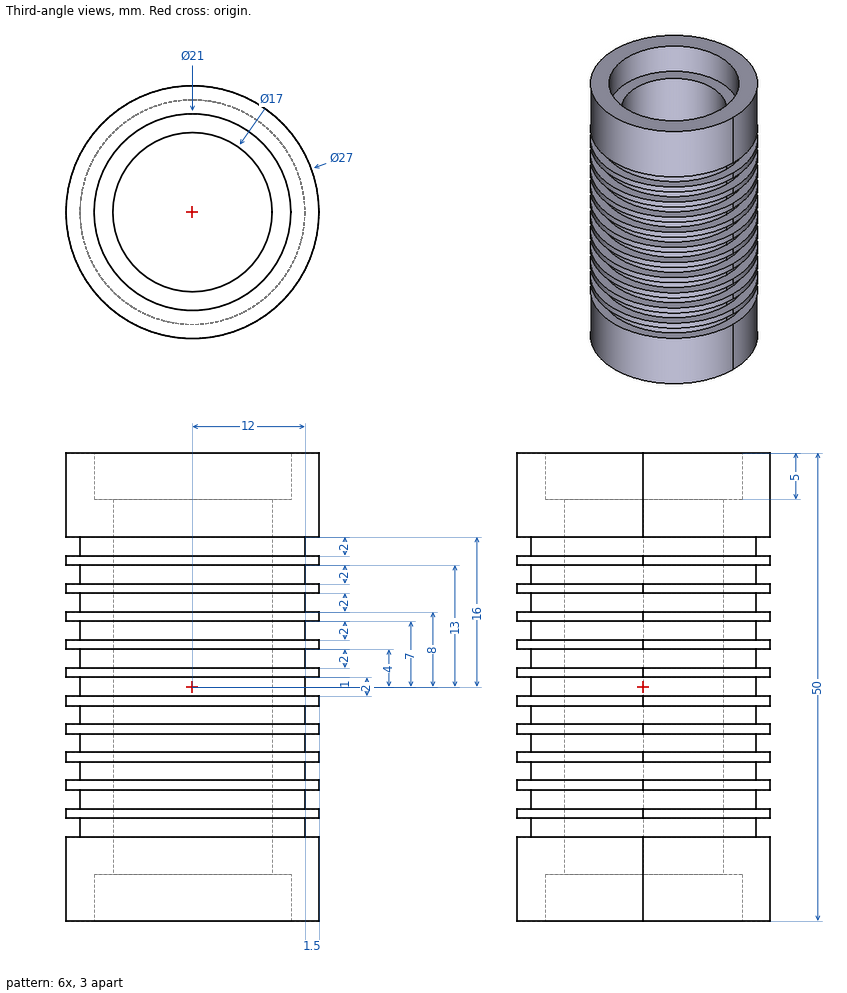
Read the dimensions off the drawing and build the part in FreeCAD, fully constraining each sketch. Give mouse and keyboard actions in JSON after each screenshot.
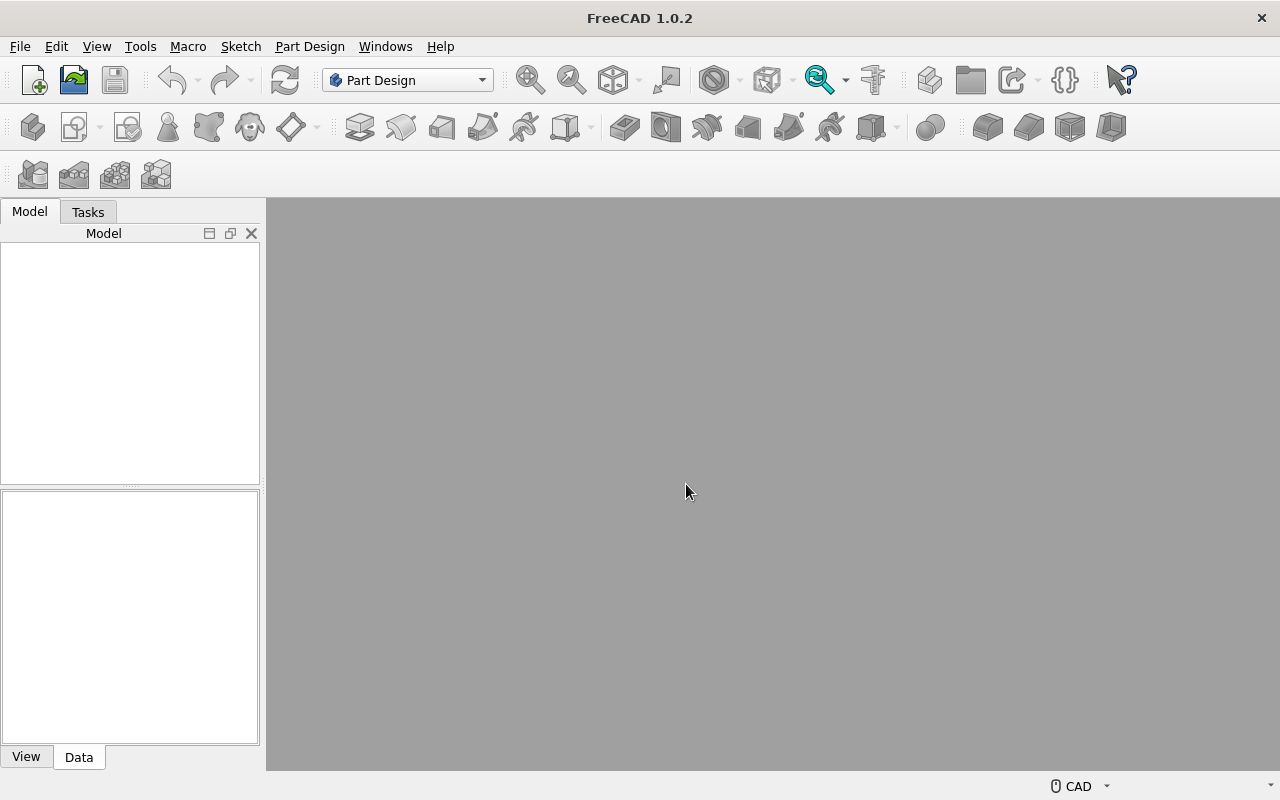
{"action": "left_click", "coordinate": [33, 80]}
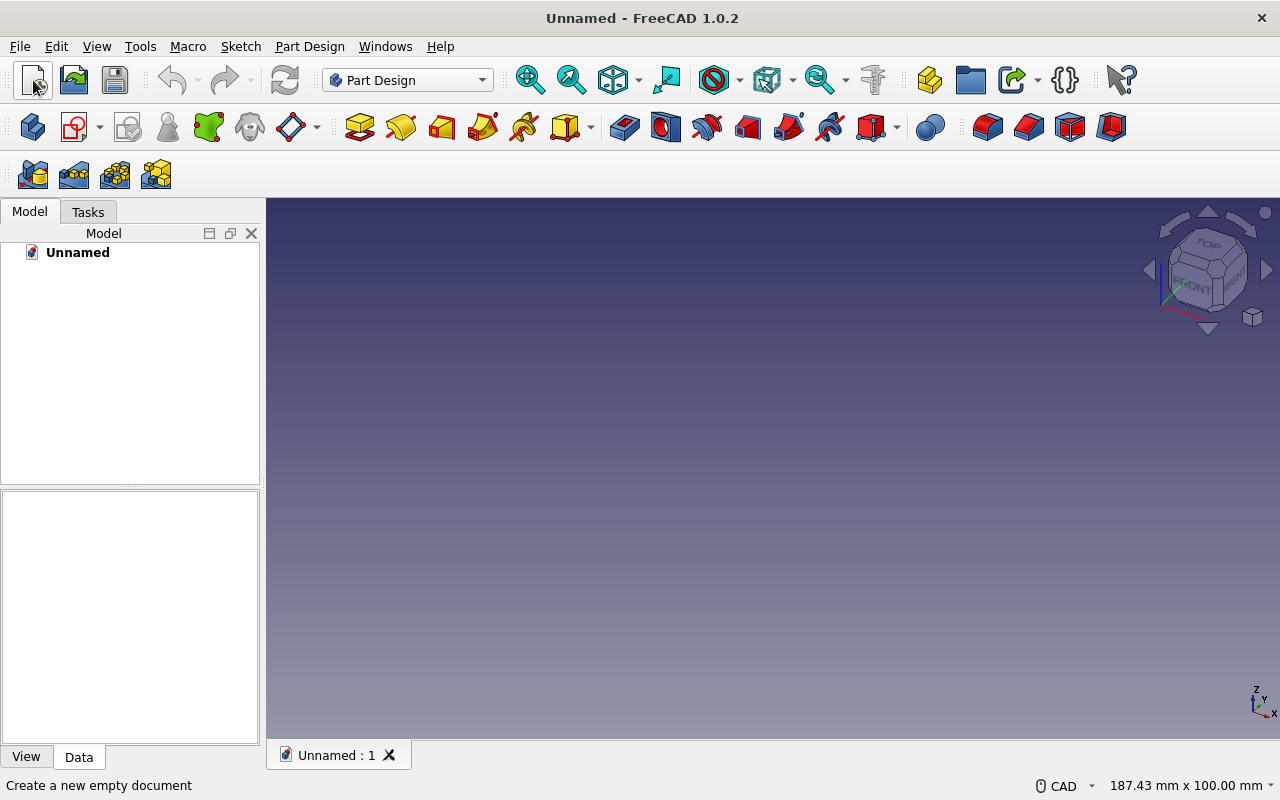
{"action": "left_click", "coordinate": [74, 128]}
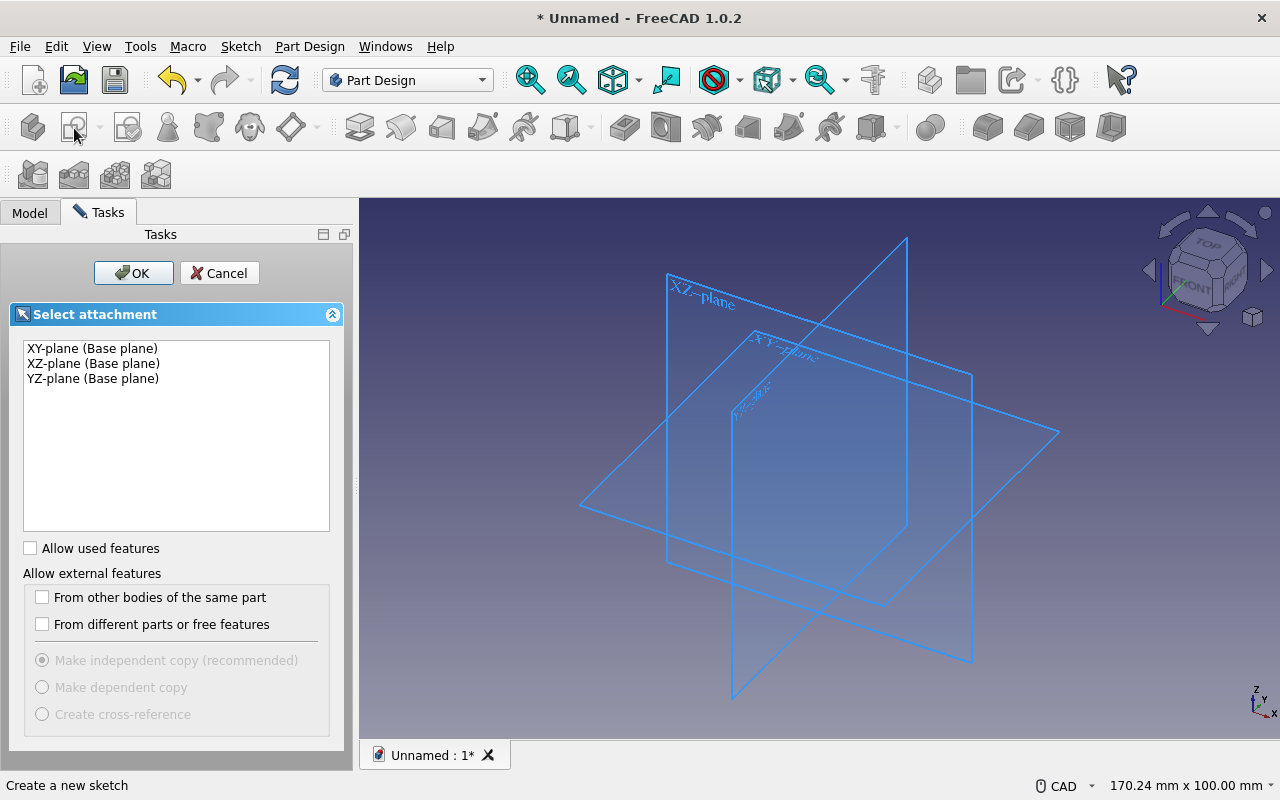
{"action": "left_click", "coordinate": [84, 348]}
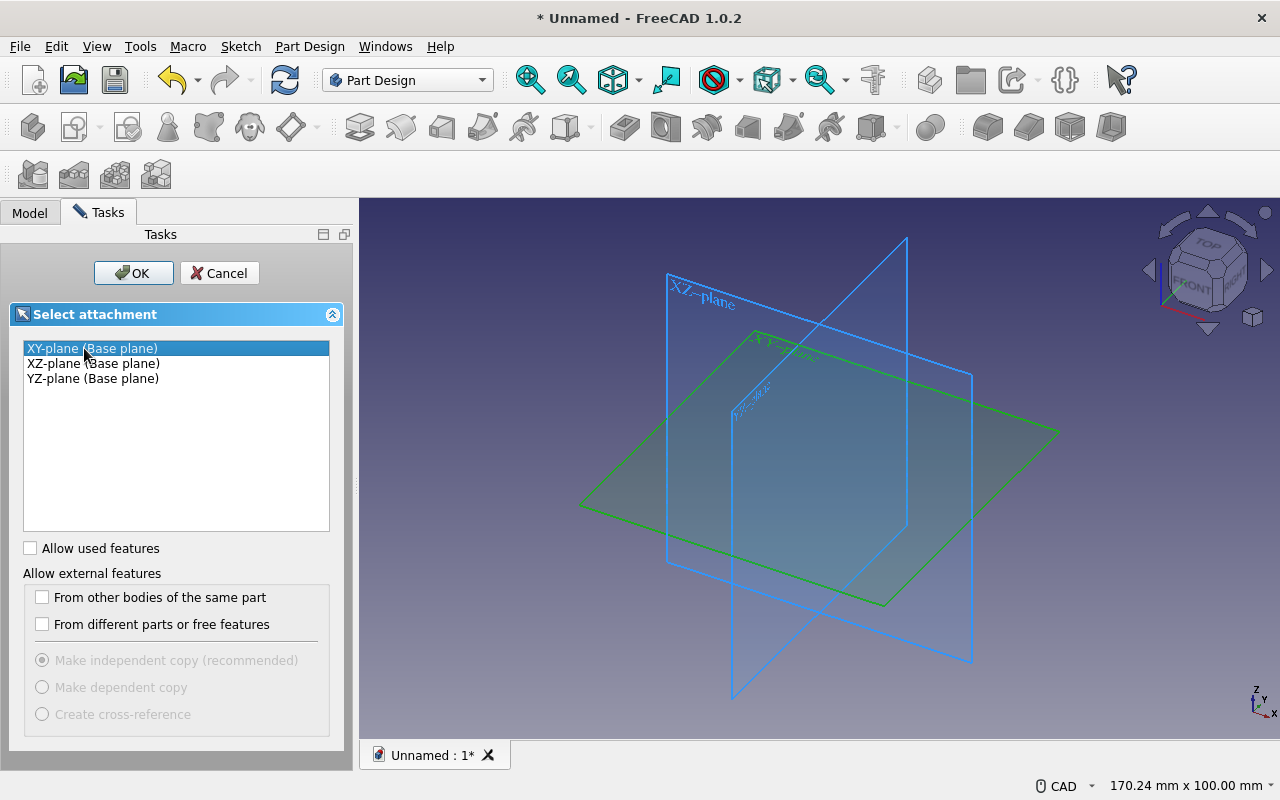
{"action": "left_click", "coordinate": [134, 273]}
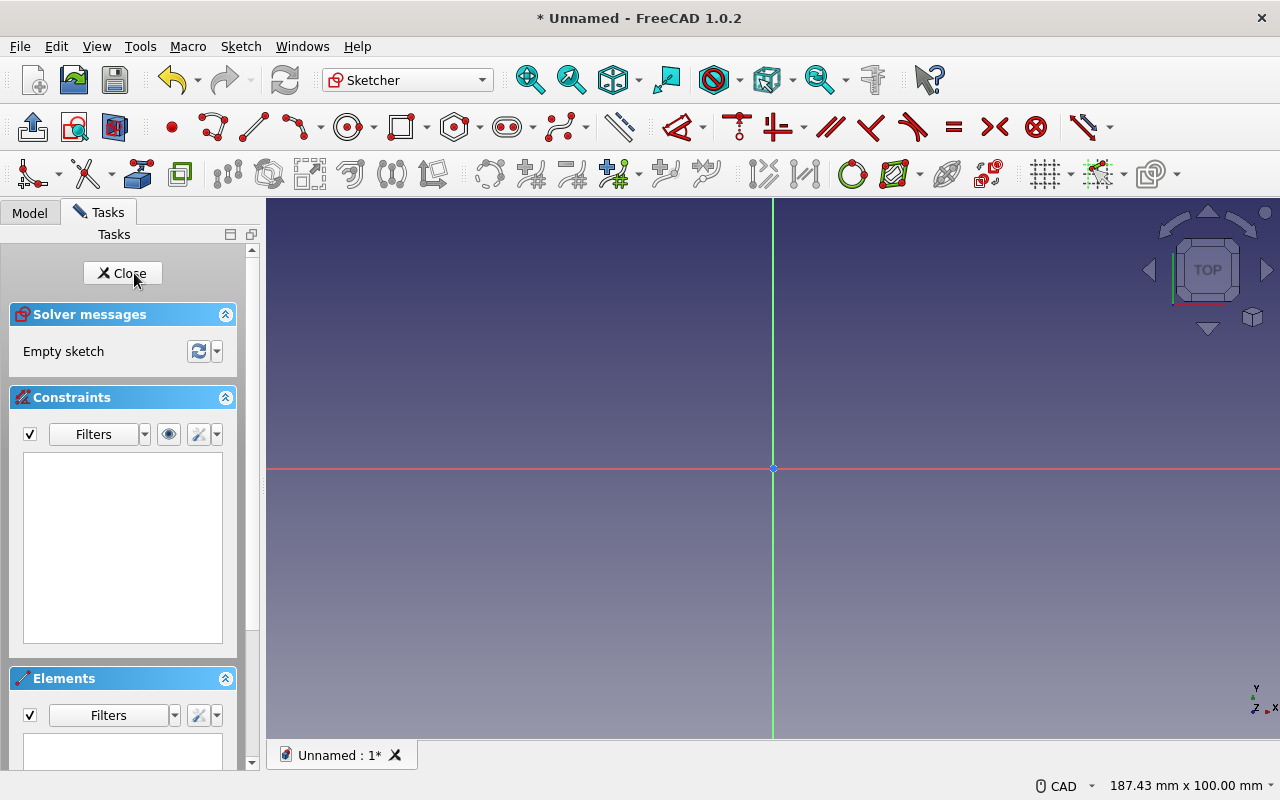
{"action": "scroll", "coordinate": [829, 469], "scroll_direction": "up", "scroll_amount": 4}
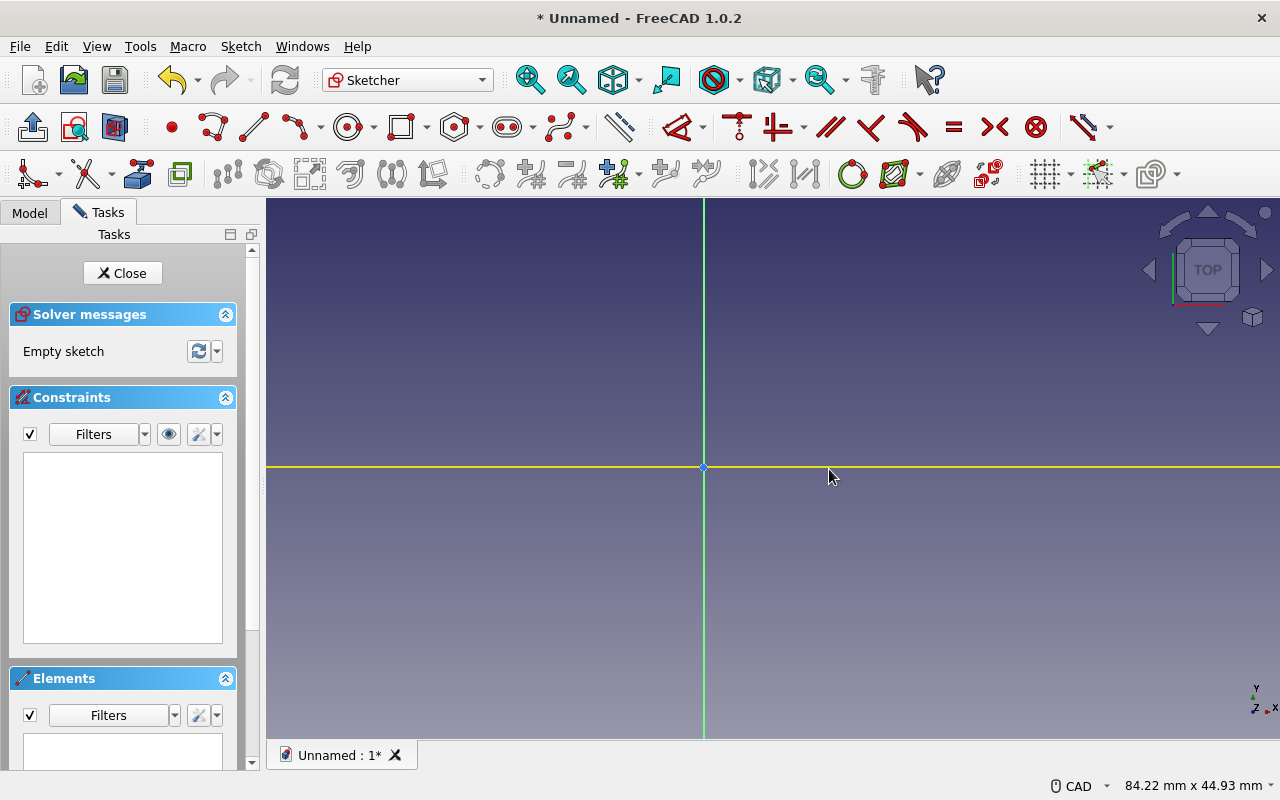
{"action": "left_click", "coordinate": [348, 128]}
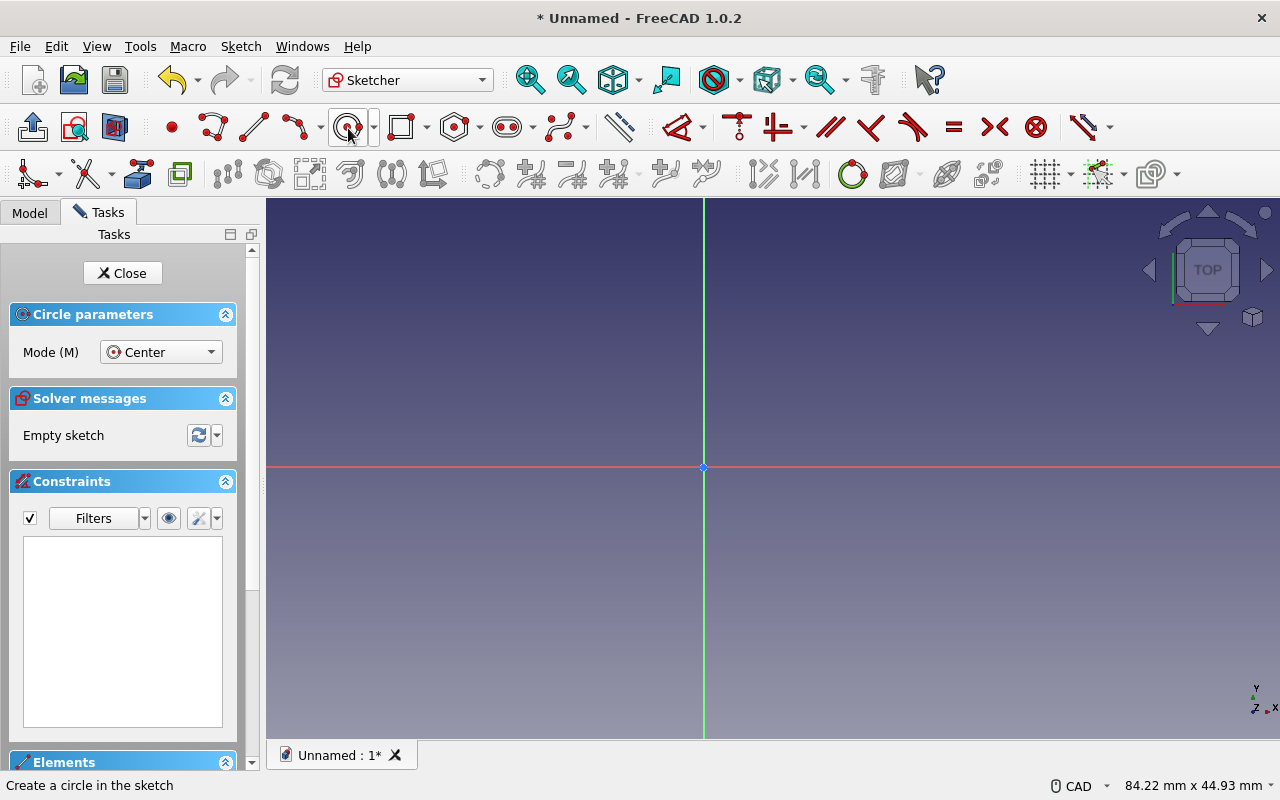
{"action": "left_click", "coordinate": [704, 467]}
{"action": "mouse_move", "coordinate": [819, 352]}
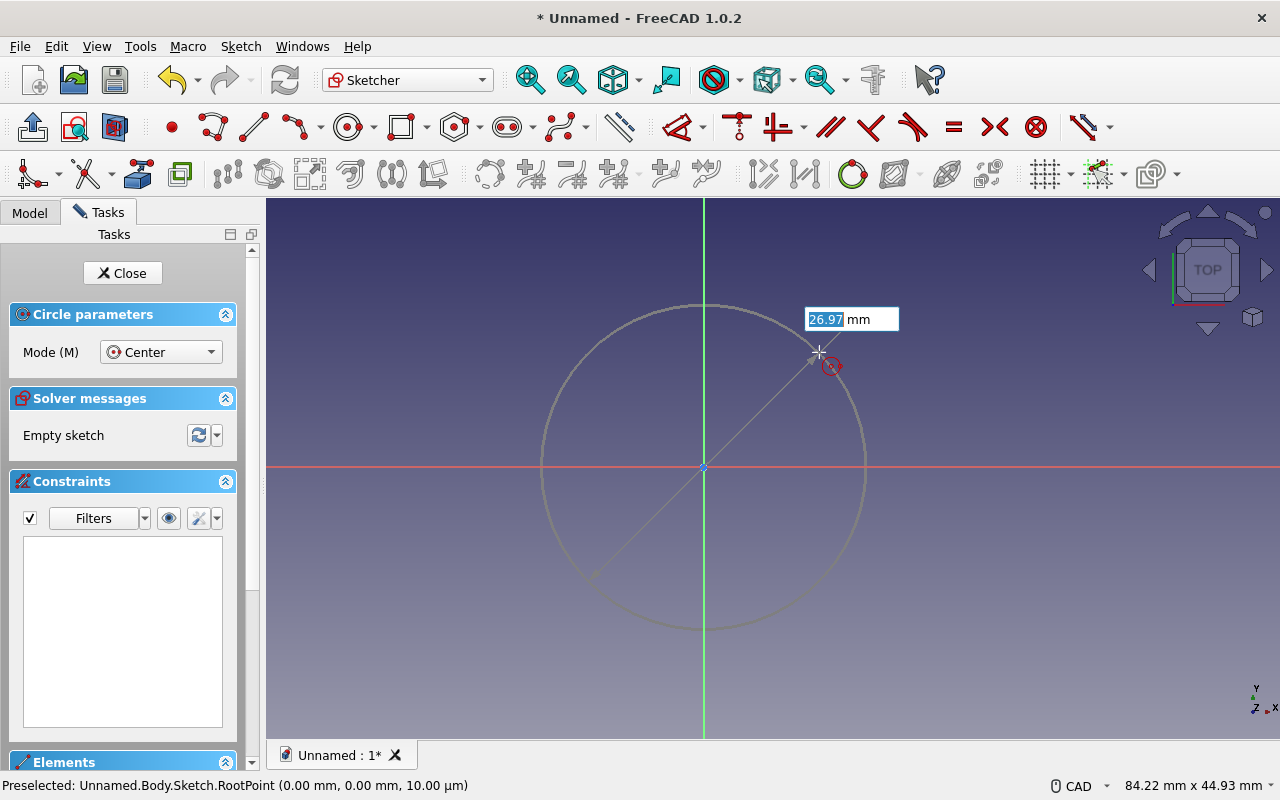
{"action": "type", "text": "27"}
{"action": "key", "text": "Return"}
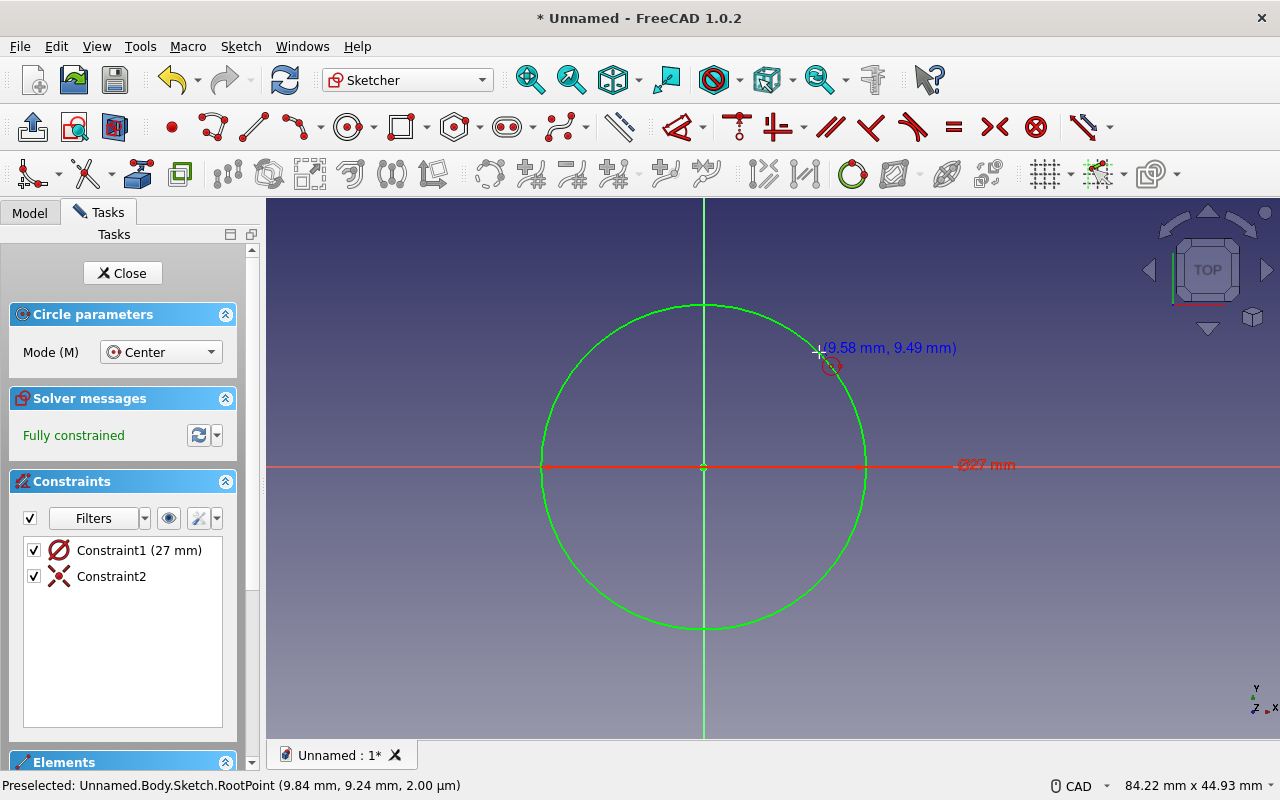
{"action": "left_click", "coordinate": [704, 467]}
{"action": "mouse_move", "coordinate": [776, 395]}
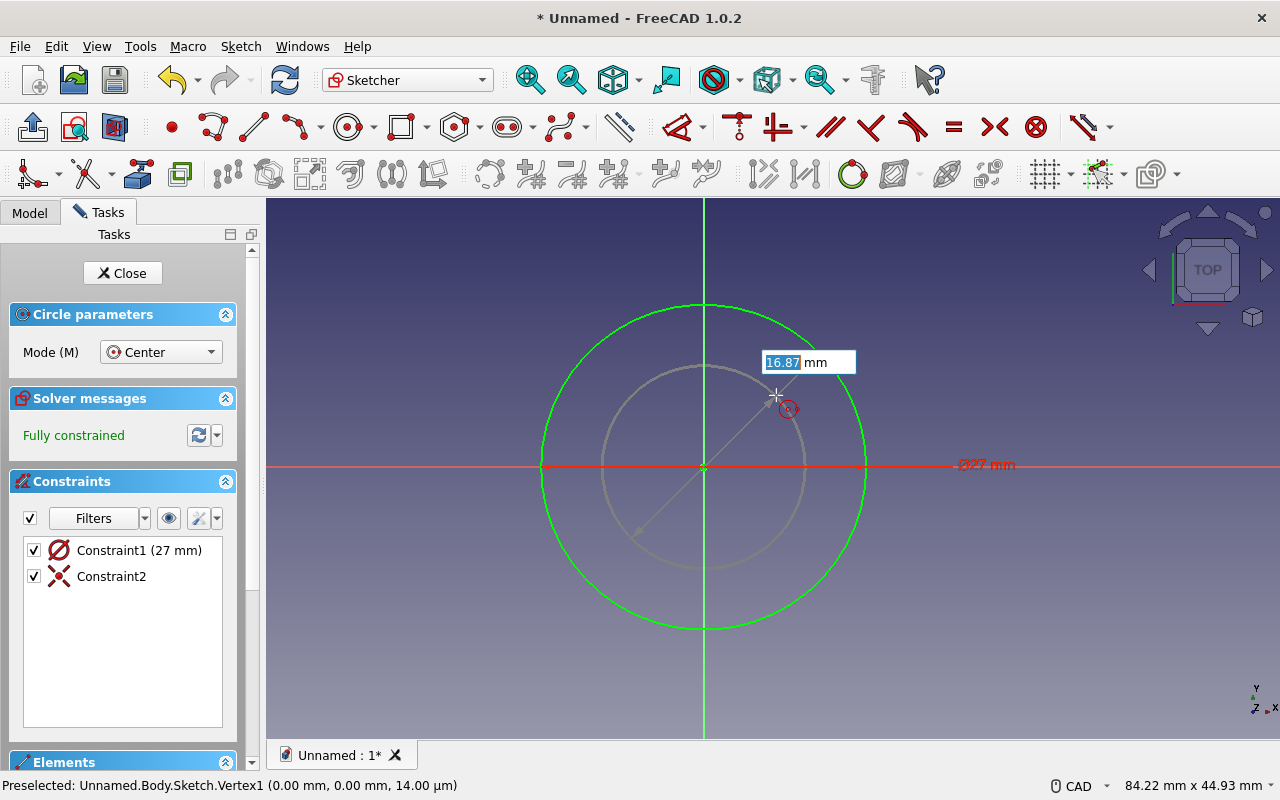
{"action": "type", "text": "17"}
{"action": "key", "text": "Return"}
{"action": "key", "text": "Escape"}